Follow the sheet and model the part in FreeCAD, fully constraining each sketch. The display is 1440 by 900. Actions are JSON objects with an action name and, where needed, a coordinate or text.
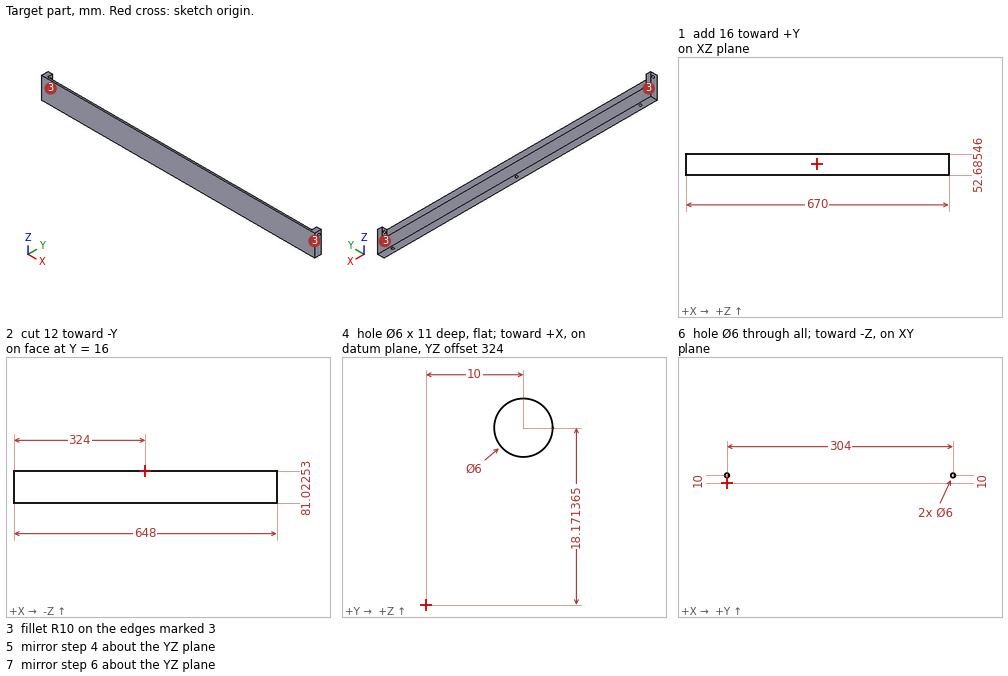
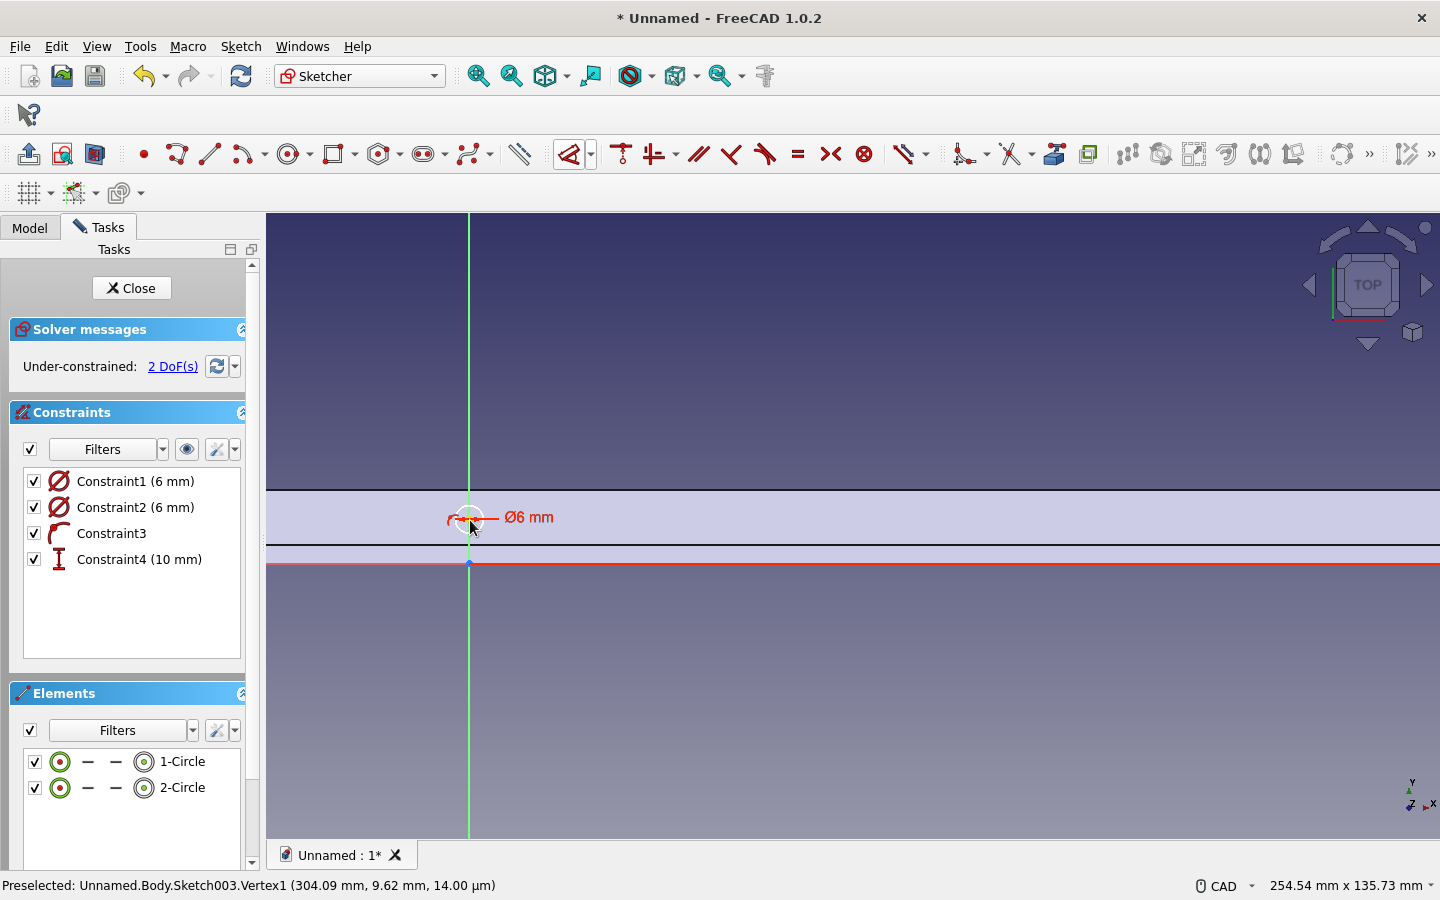
{"action": "left_click", "coordinate": [469, 519]}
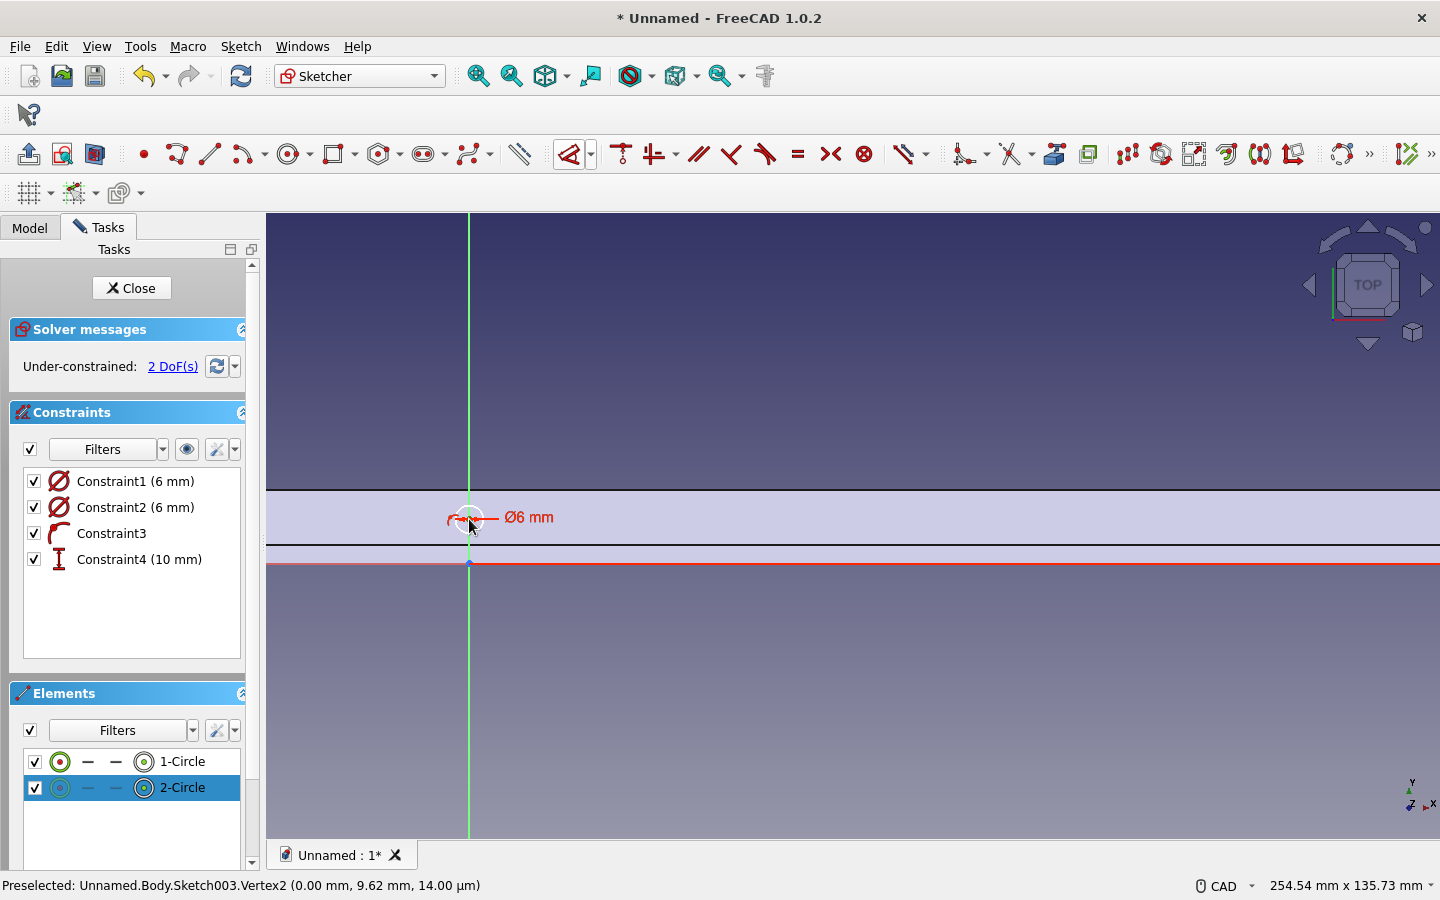
{"action": "key", "text": "i"}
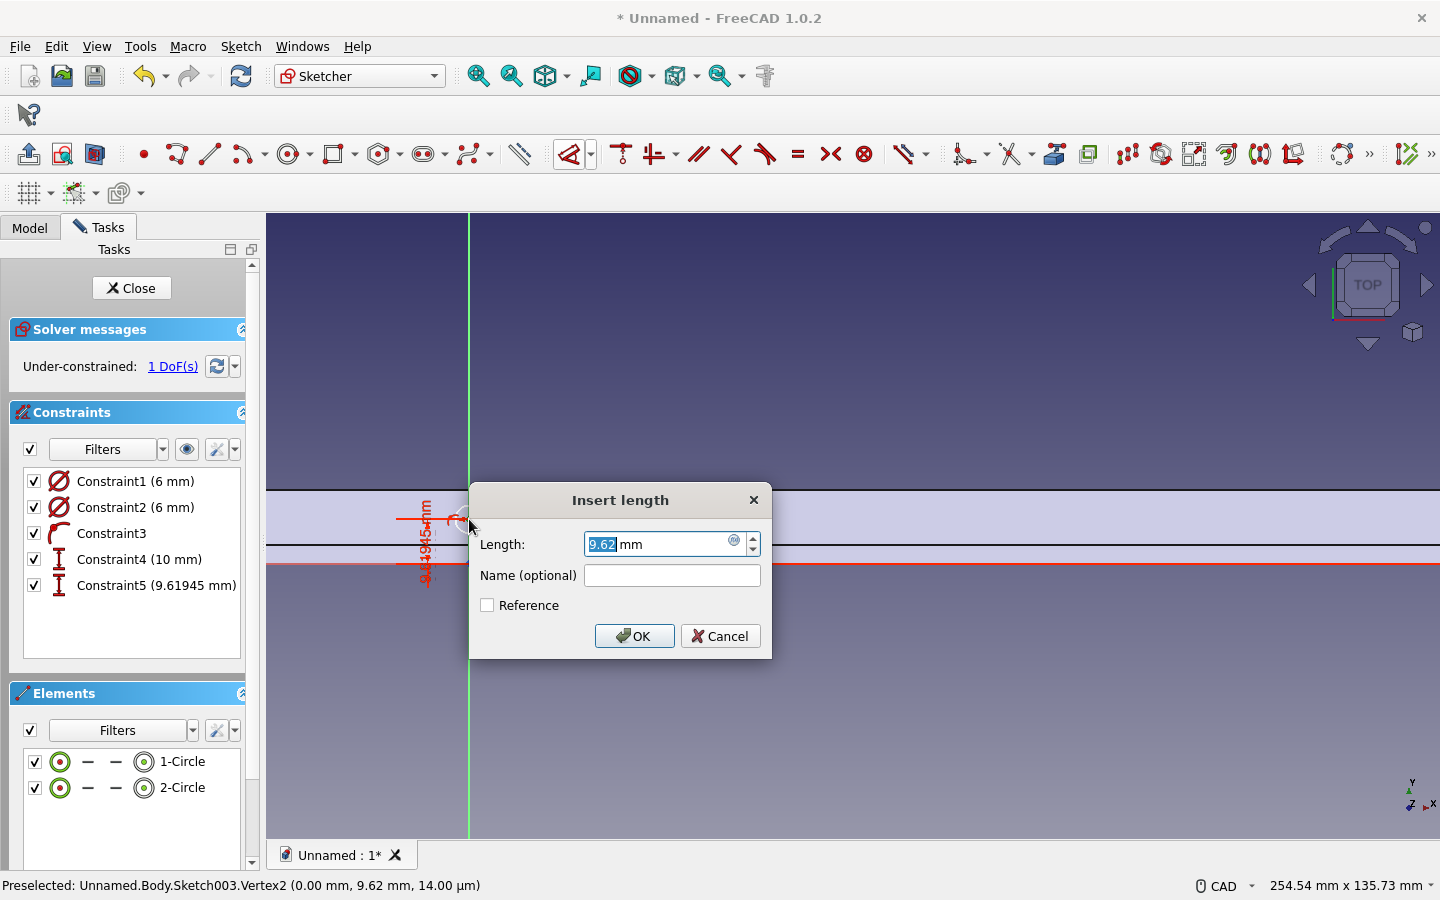
{"action": "type", "text": "10"}
{"action": "key", "text": "Return"}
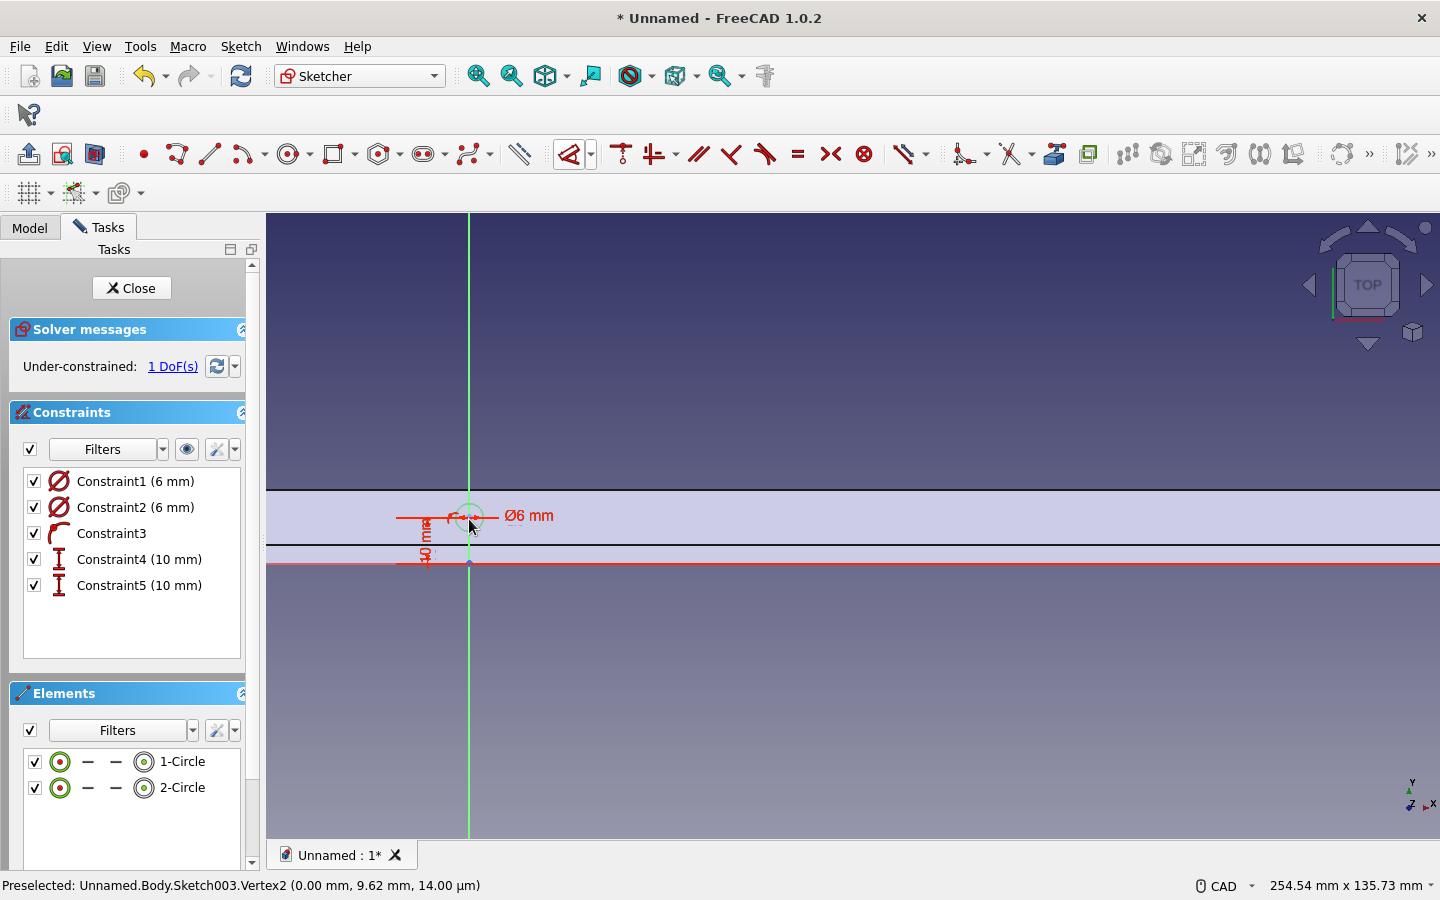
{"action": "scroll", "coordinate": [470, 520], "scroll_direction": "down", "scroll_amount": 4}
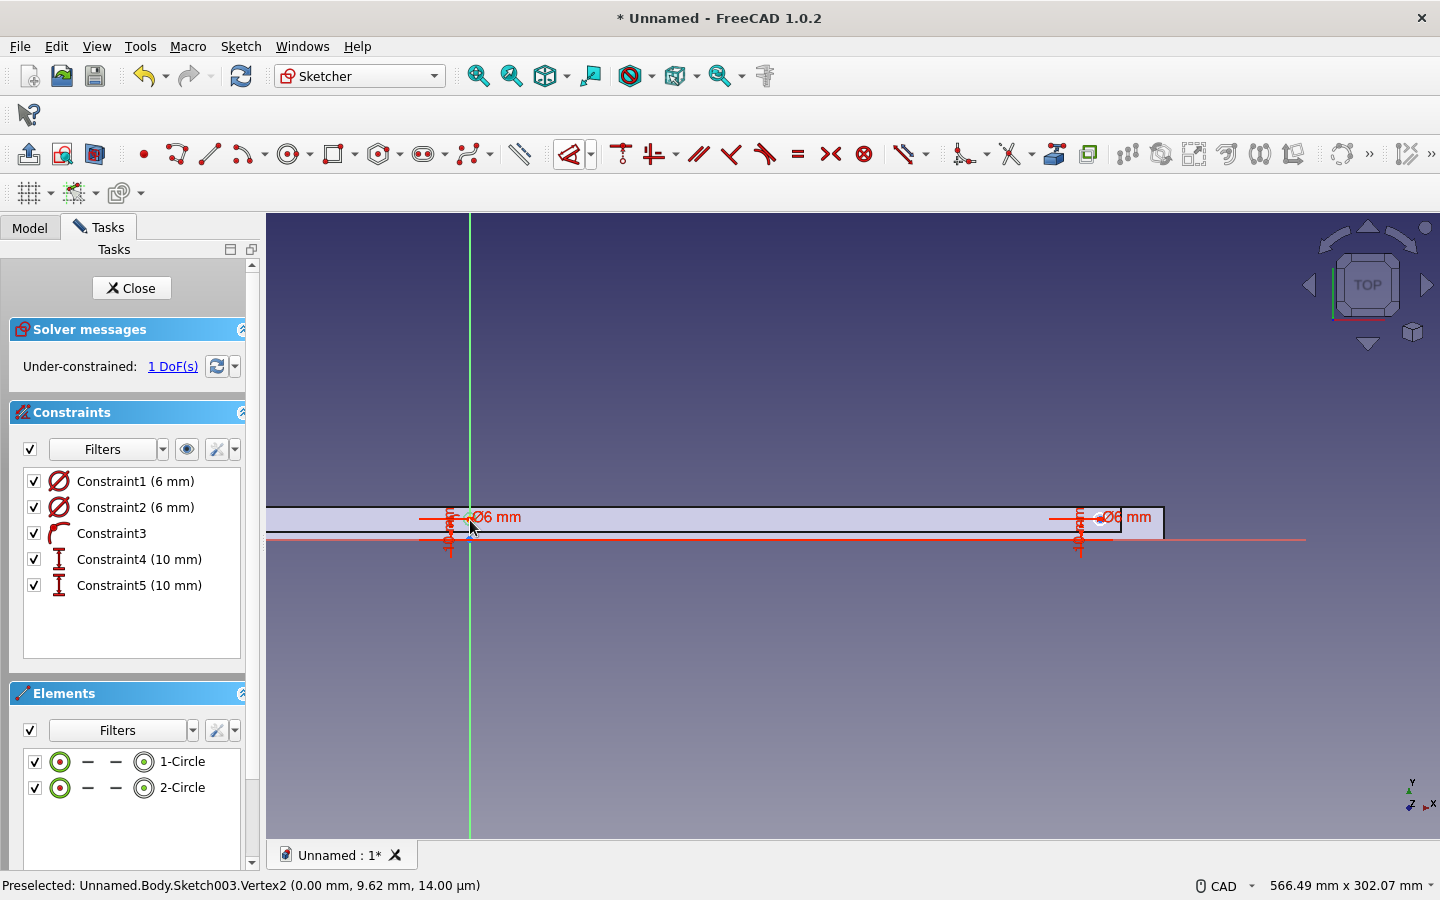
{"action": "left_click", "coordinate": [1100, 519]}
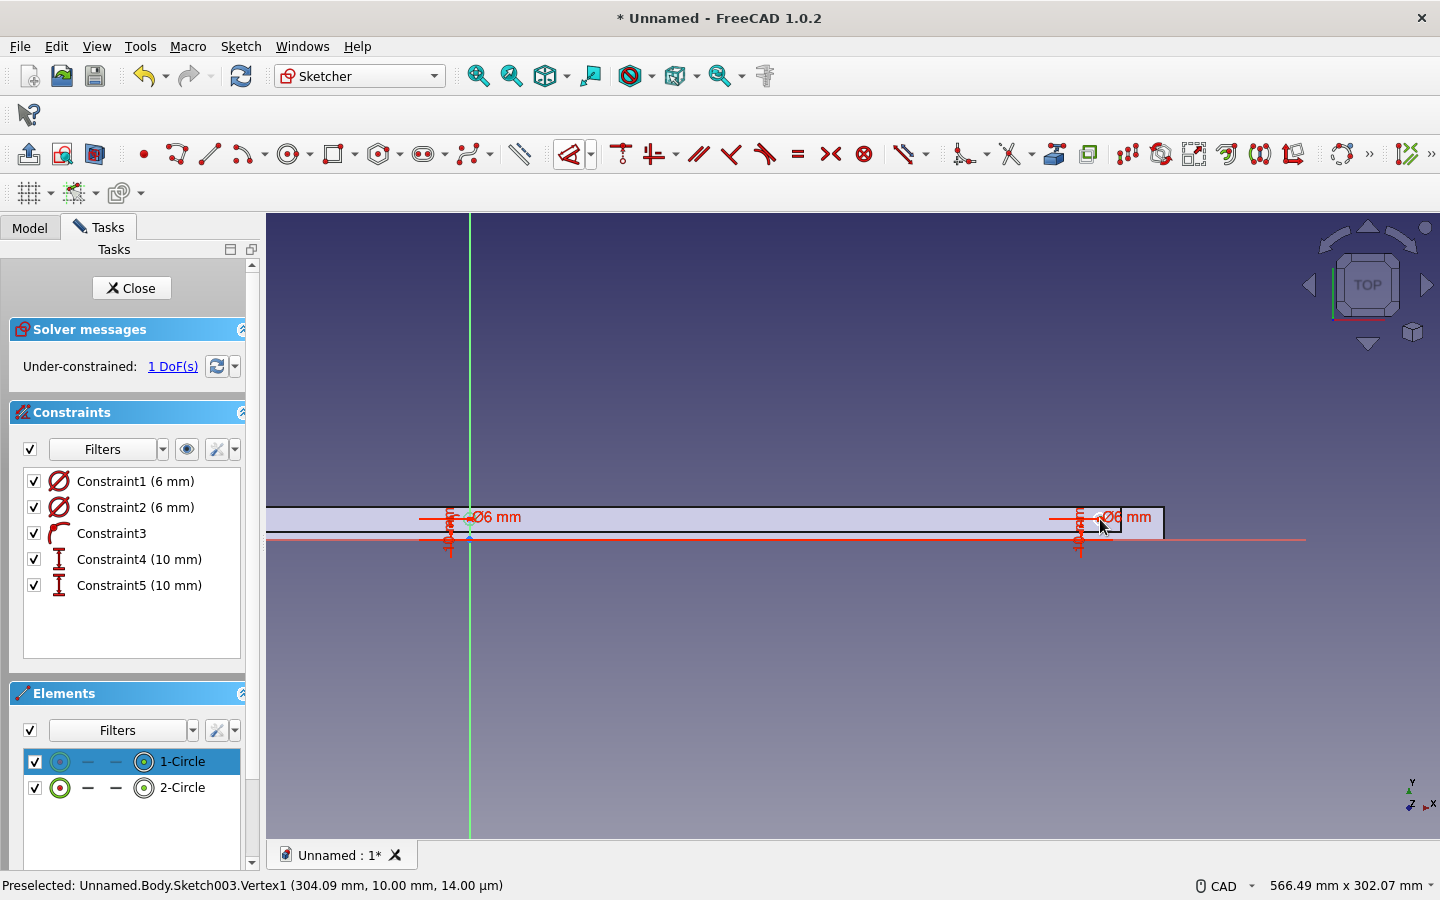
{"action": "left_click", "coordinate": [590, 154]}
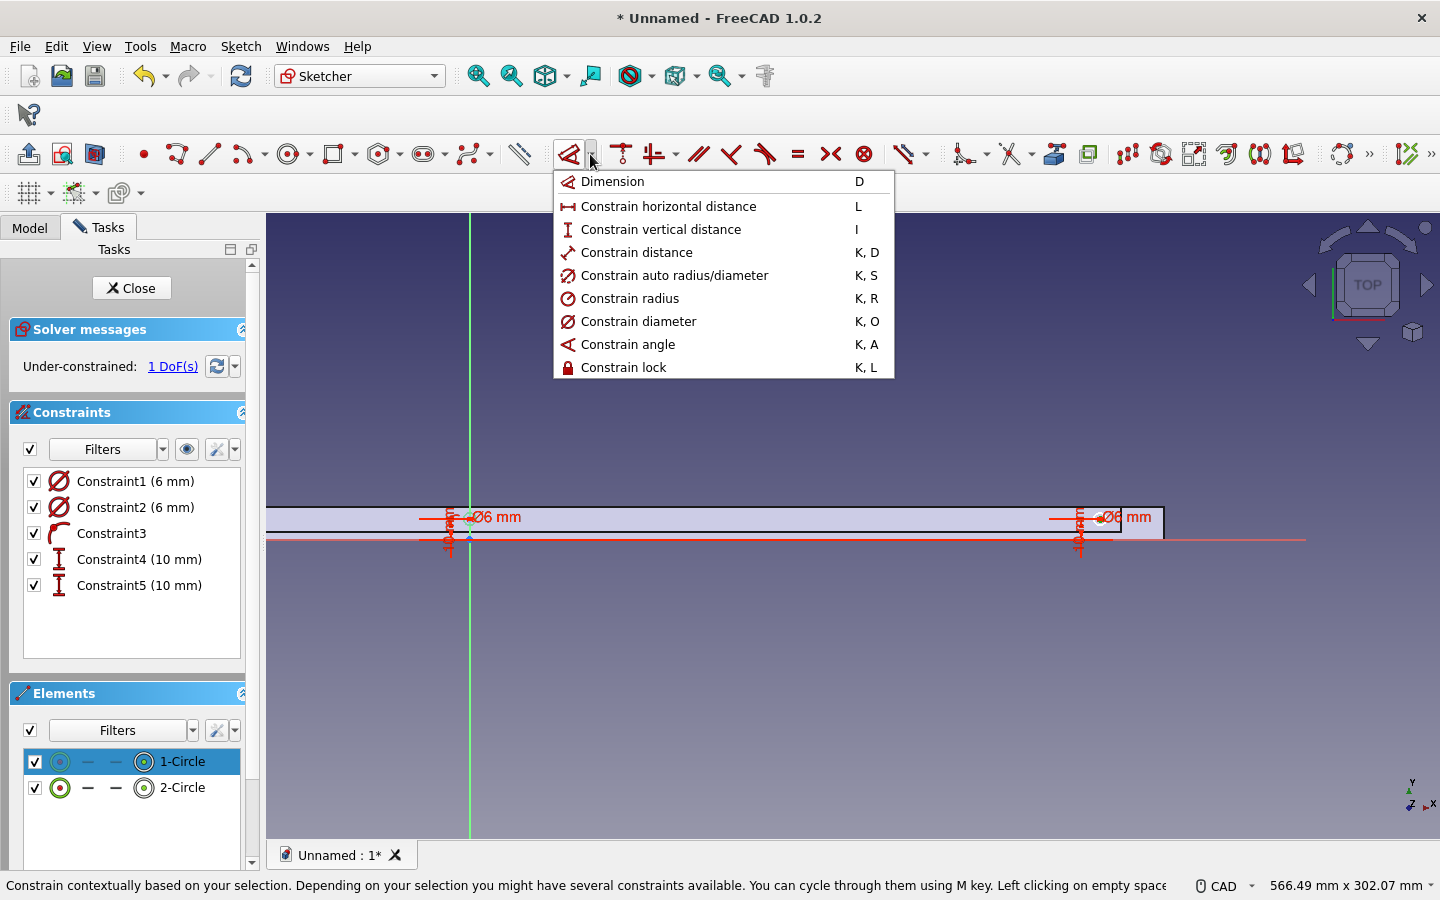
{"action": "left_click", "coordinate": [724, 206]}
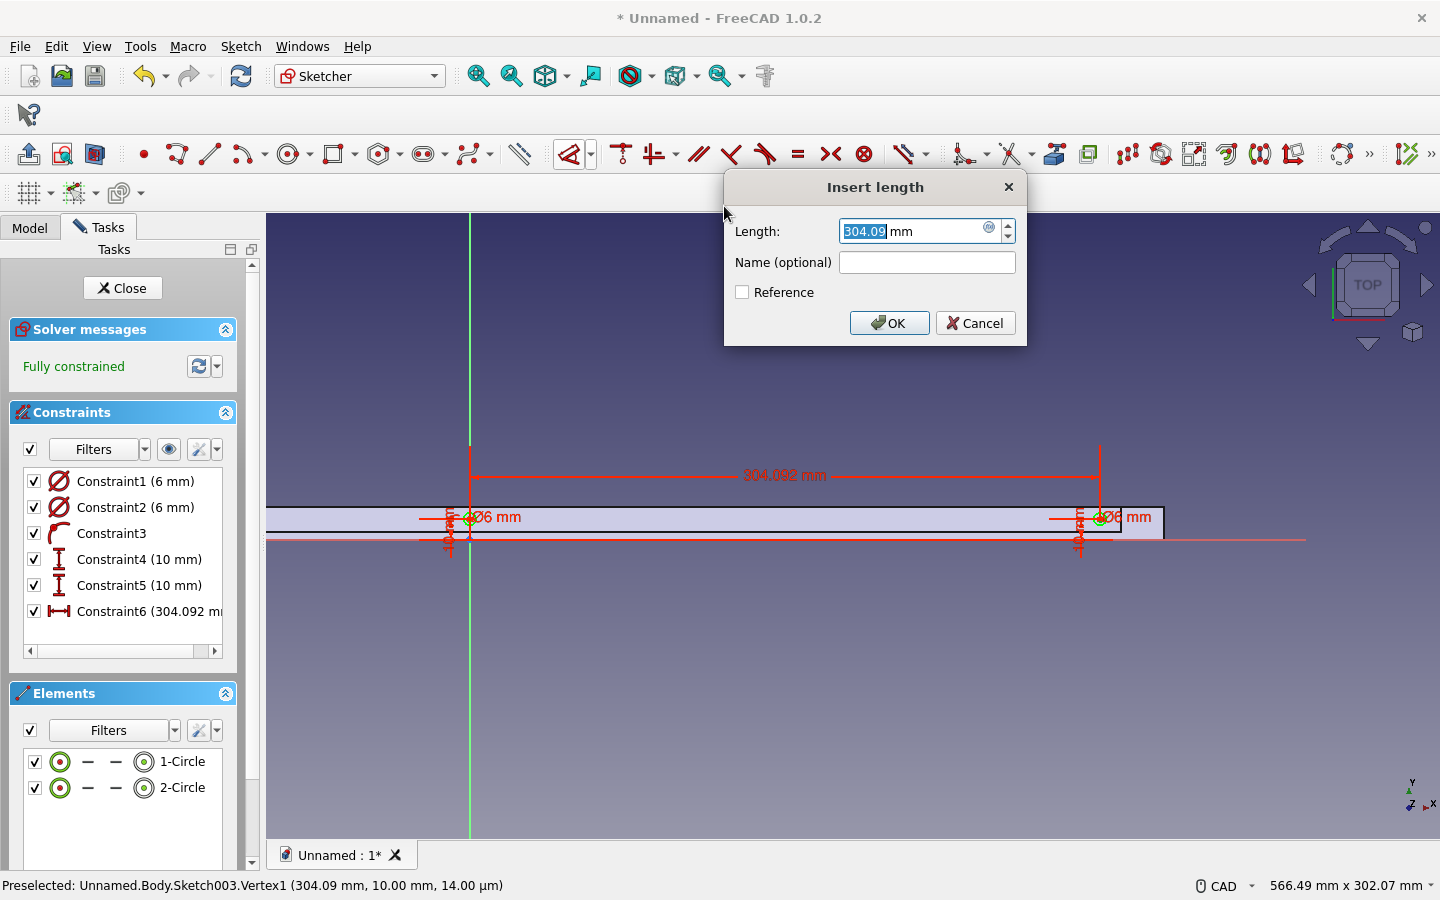
{"action": "type", "text": "304"}
{"action": "key", "text": "Return"}